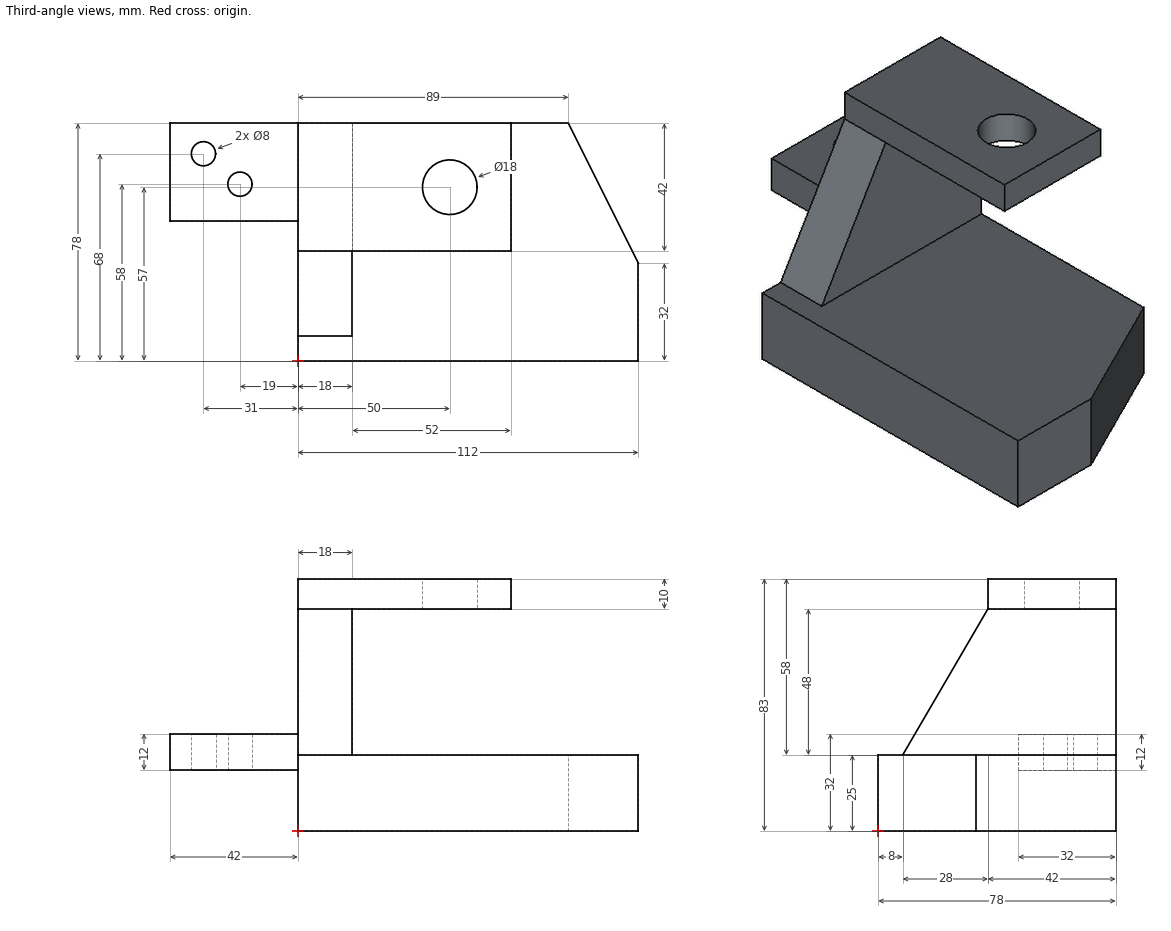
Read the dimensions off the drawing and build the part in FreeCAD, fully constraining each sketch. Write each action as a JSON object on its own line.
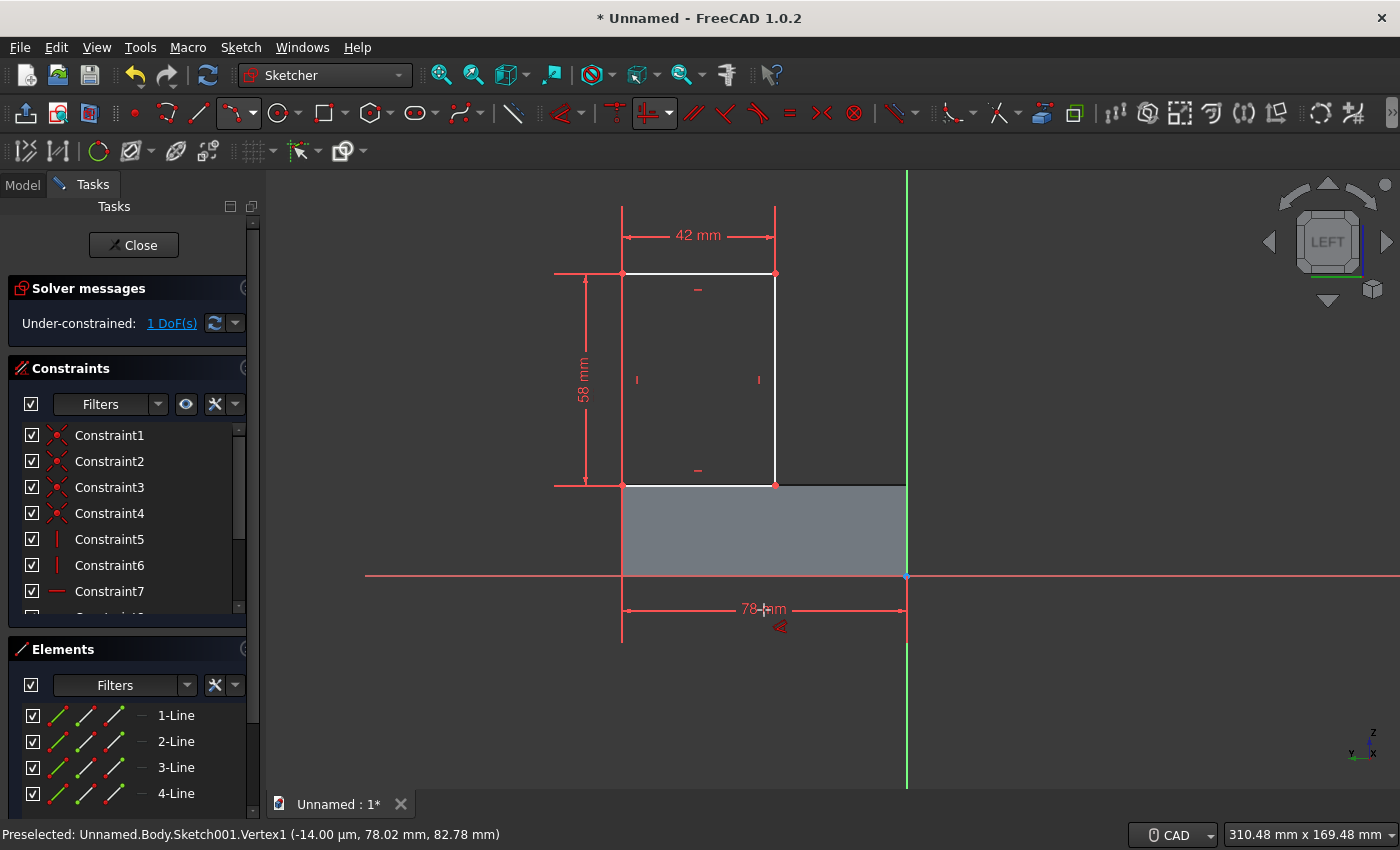
{"action": "left_click", "coordinate": [622, 274]}
{"action": "left_click", "coordinate": [941, 425]}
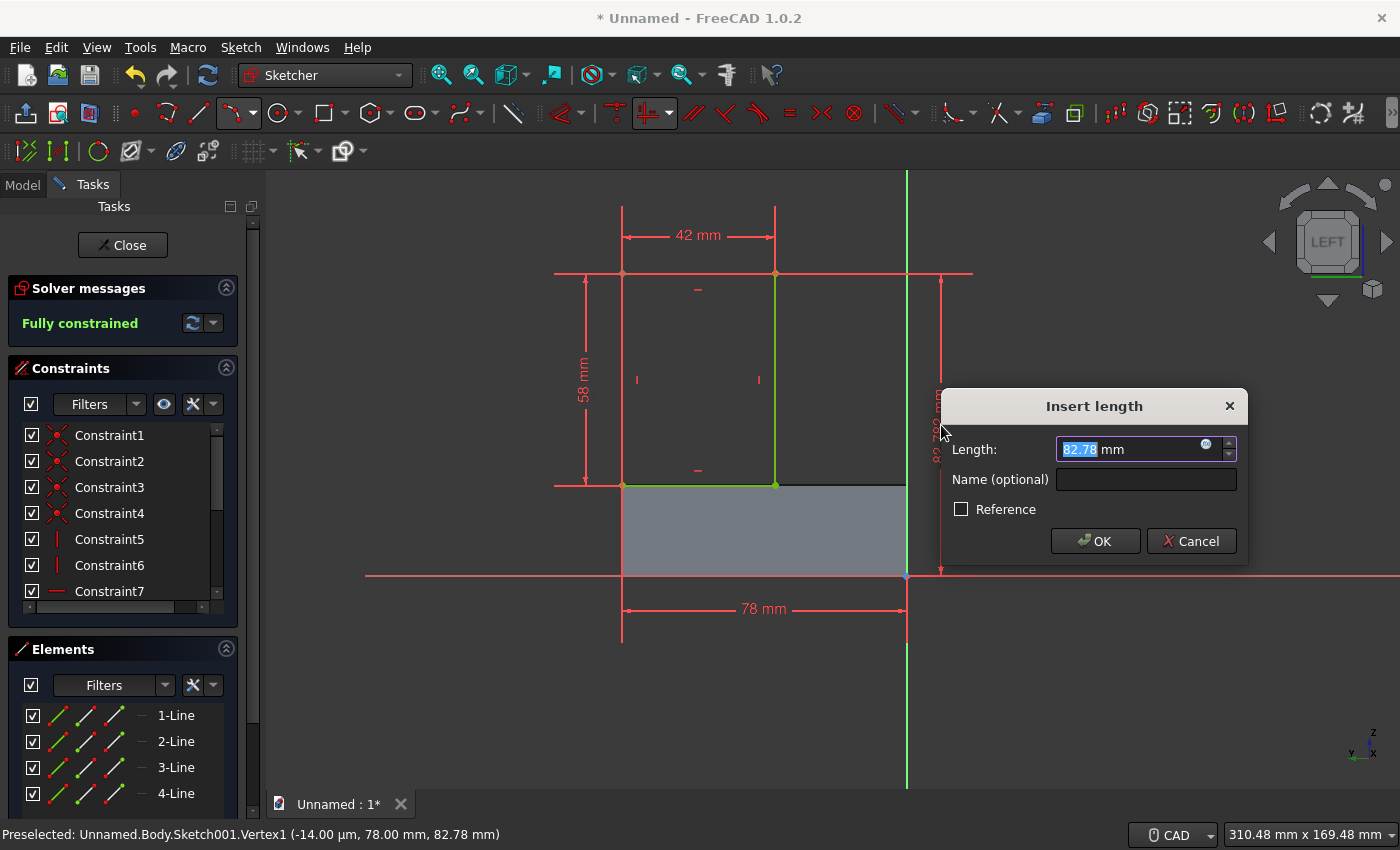
{"action": "type", "text": "83"}
{"action": "key", "text": "Return"}
{"action": "key", "text": "Escape"}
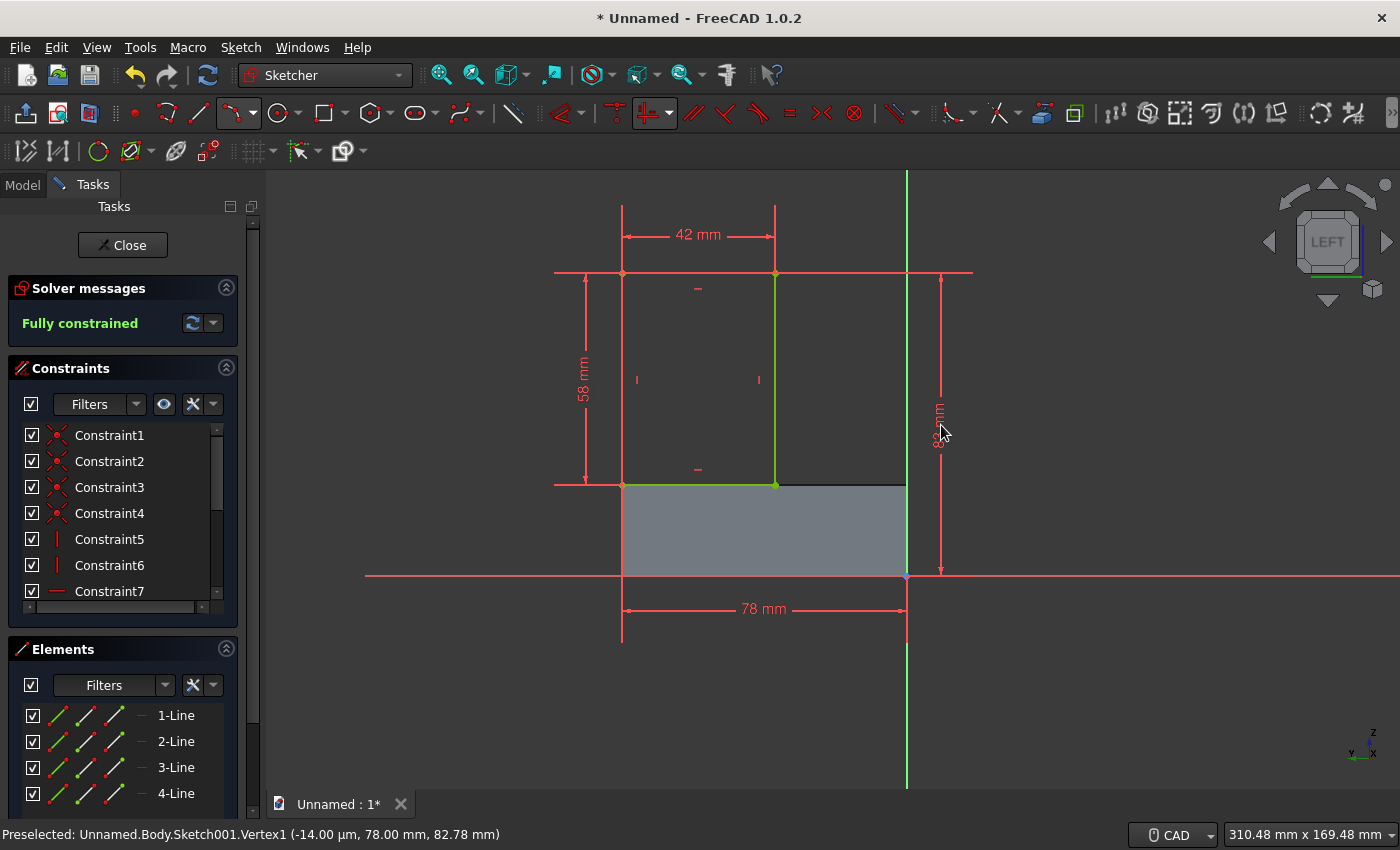
{"action": "left_click", "coordinate": [123, 245]}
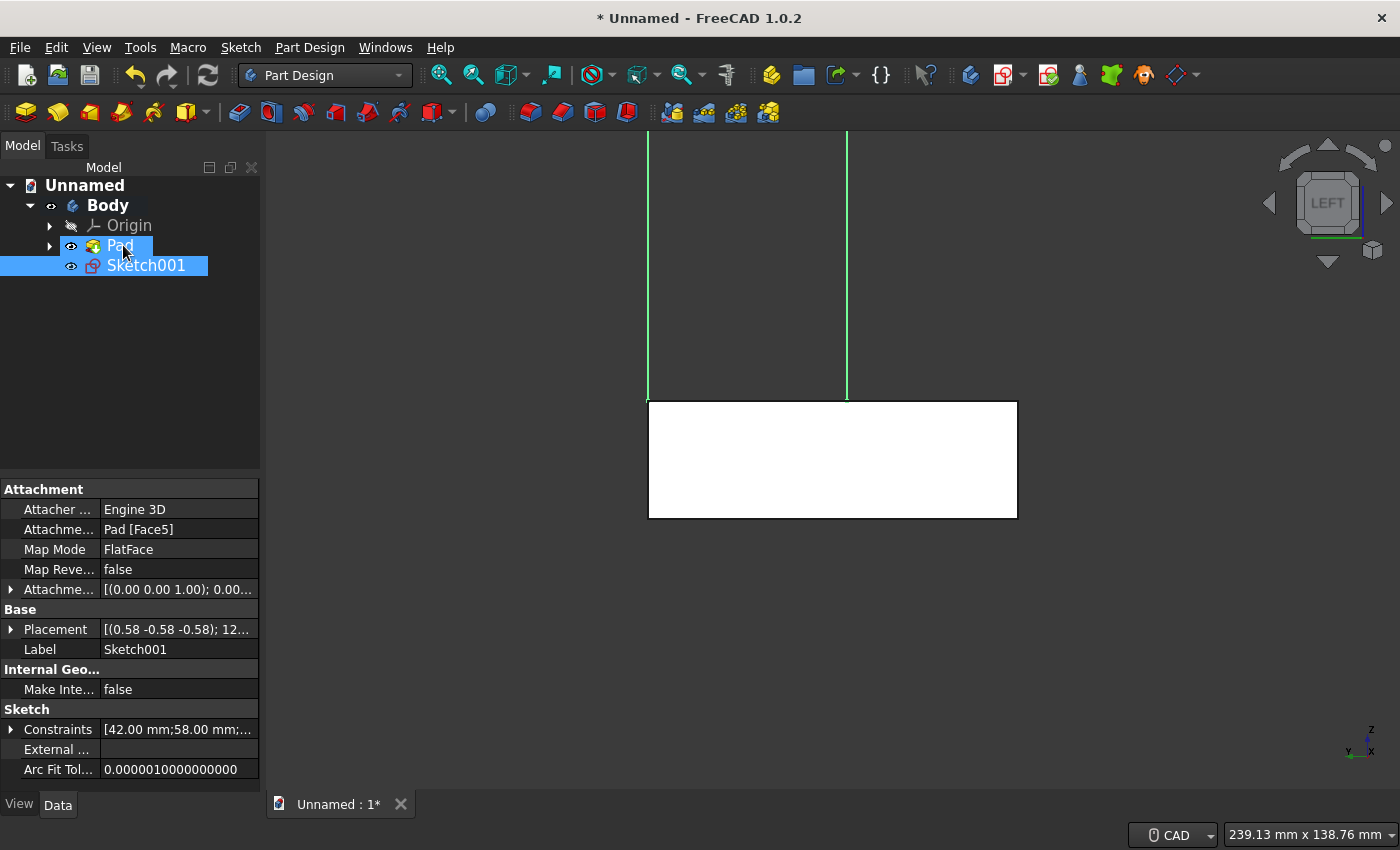
{"action": "left_click", "coordinate": [26, 112]}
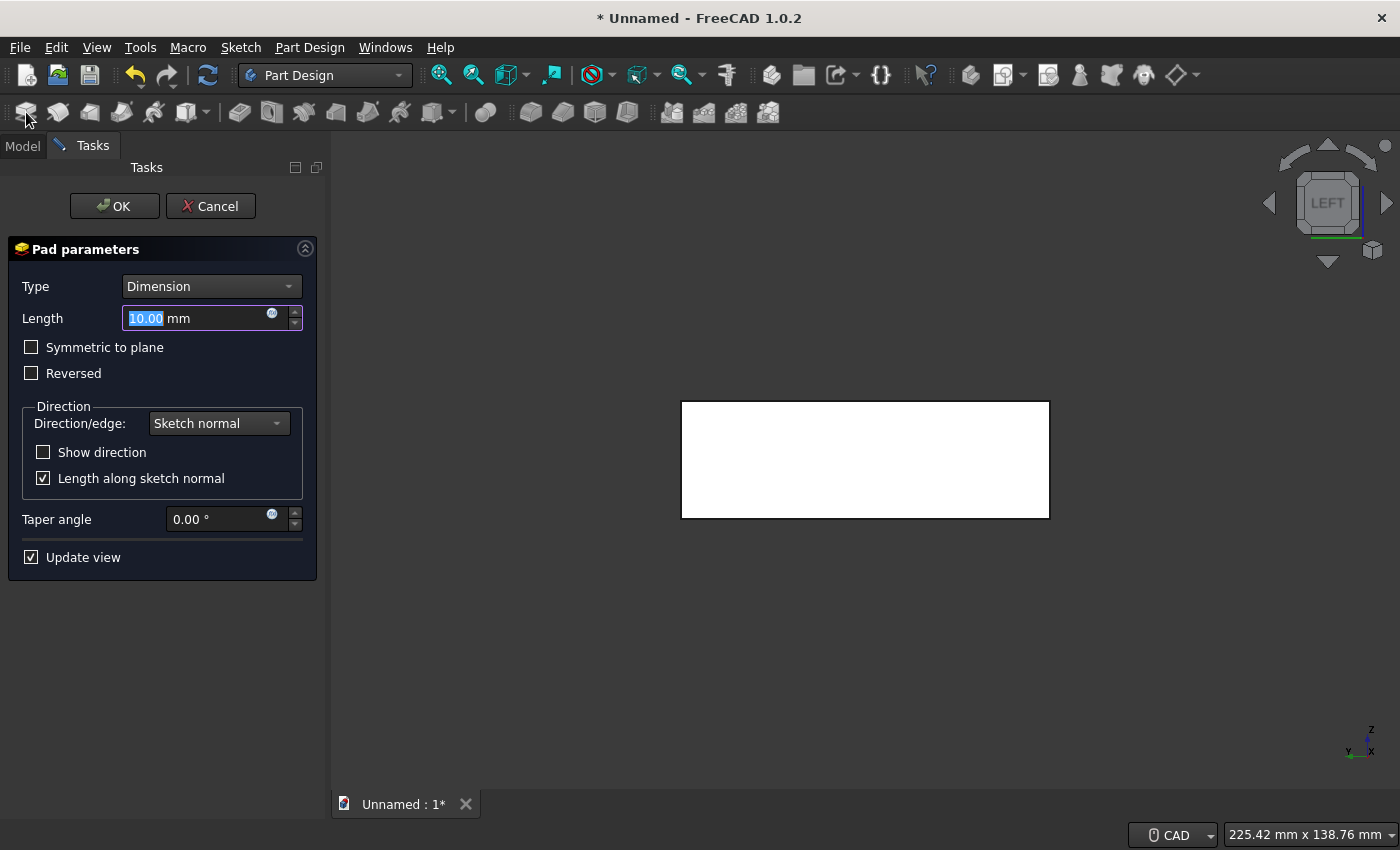
{"action": "type", "text": "18"}
{"action": "key", "text": "Tab"}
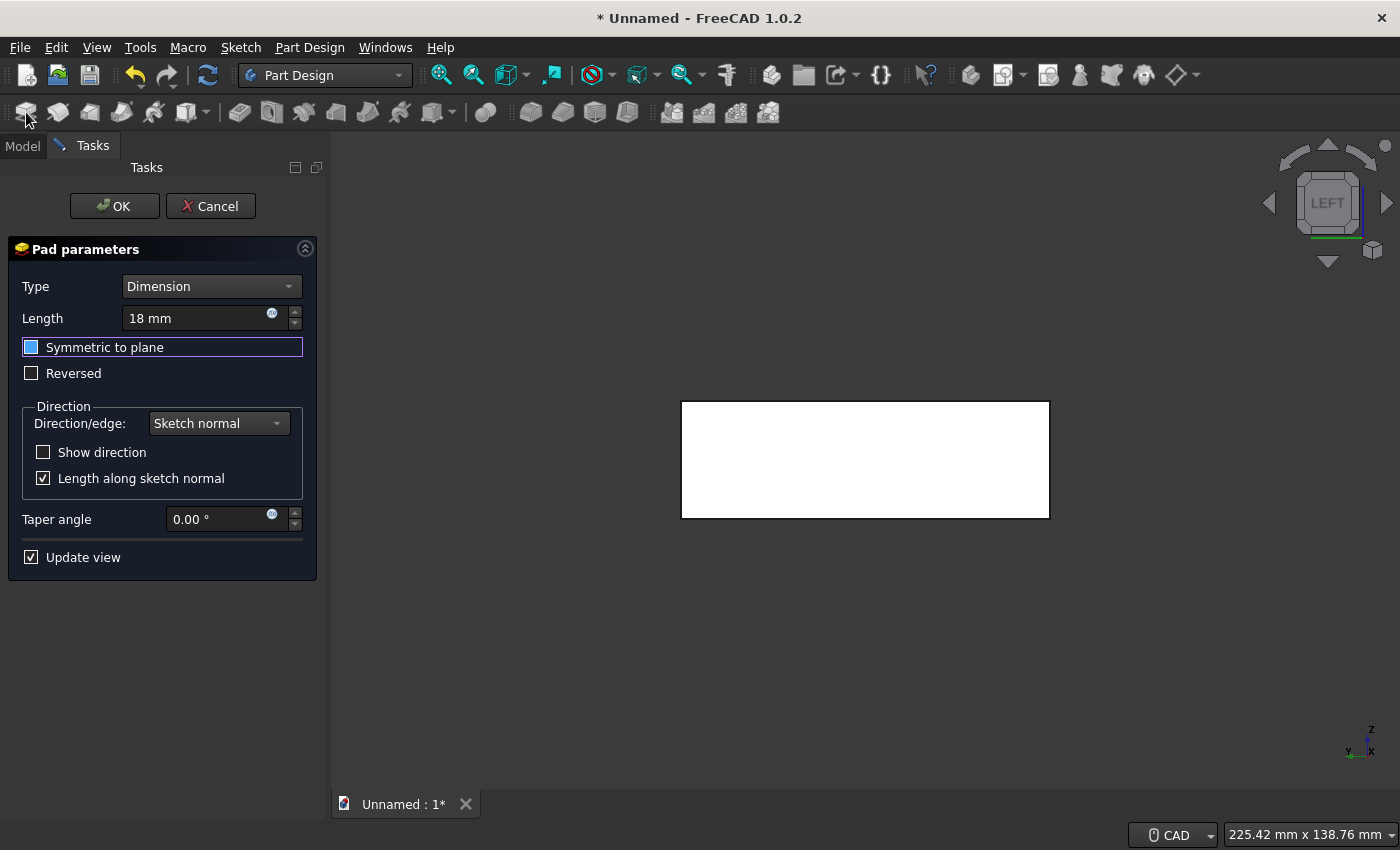
{"action": "left_click", "coordinate": [30, 373]}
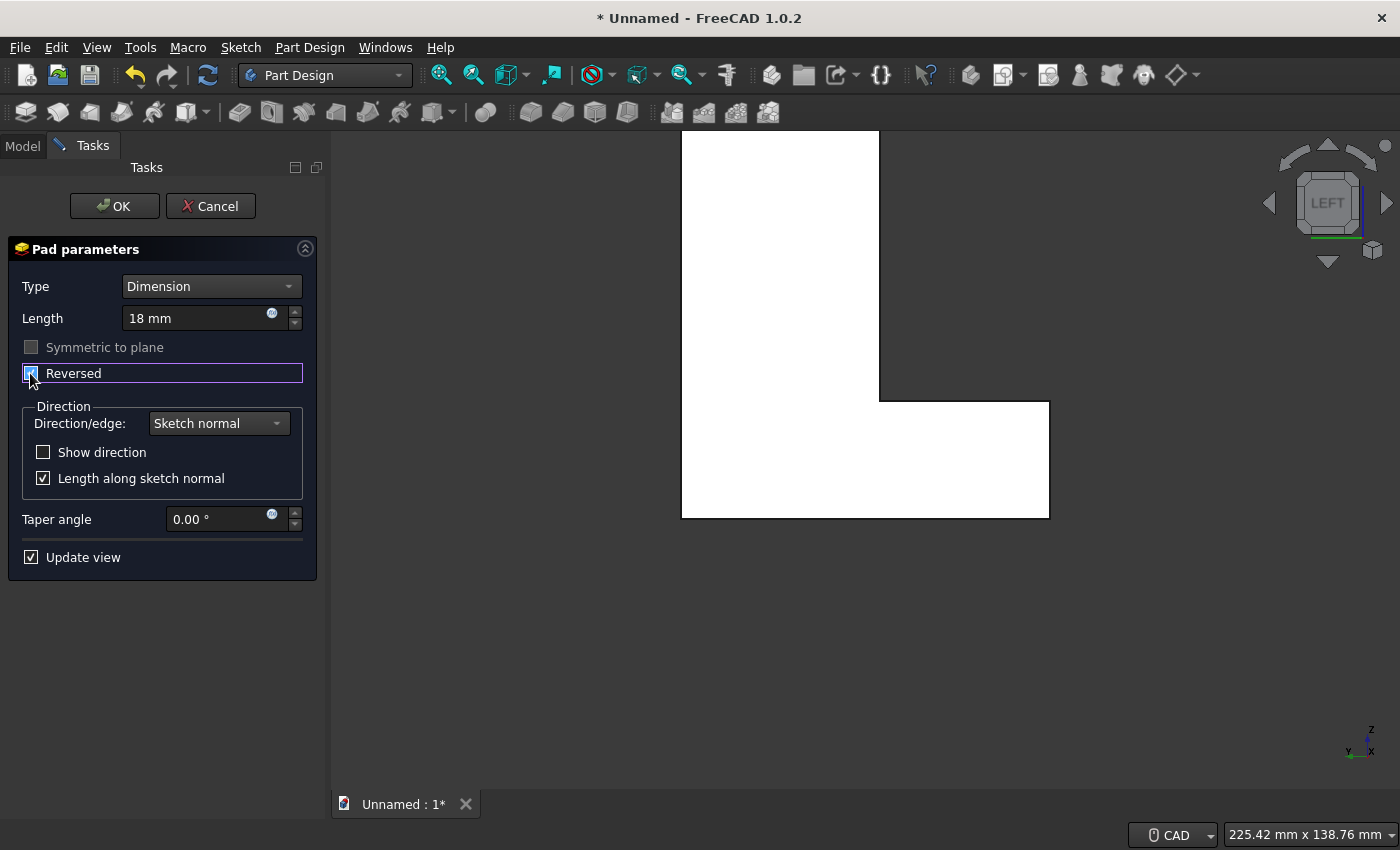
{"action": "left_click", "coordinate": [115, 206]}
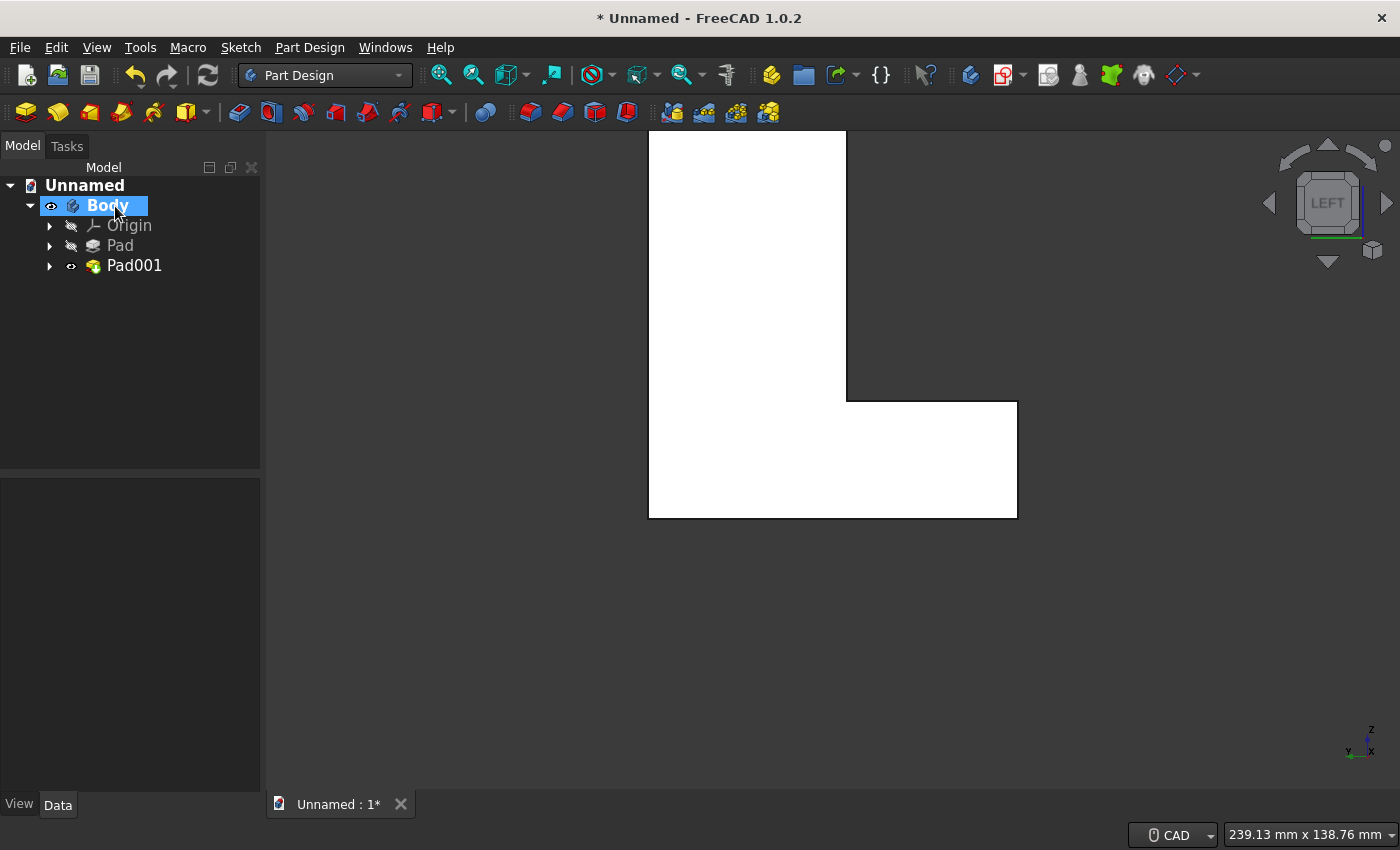
{"action": "left_click", "coordinate": [442, 76]}